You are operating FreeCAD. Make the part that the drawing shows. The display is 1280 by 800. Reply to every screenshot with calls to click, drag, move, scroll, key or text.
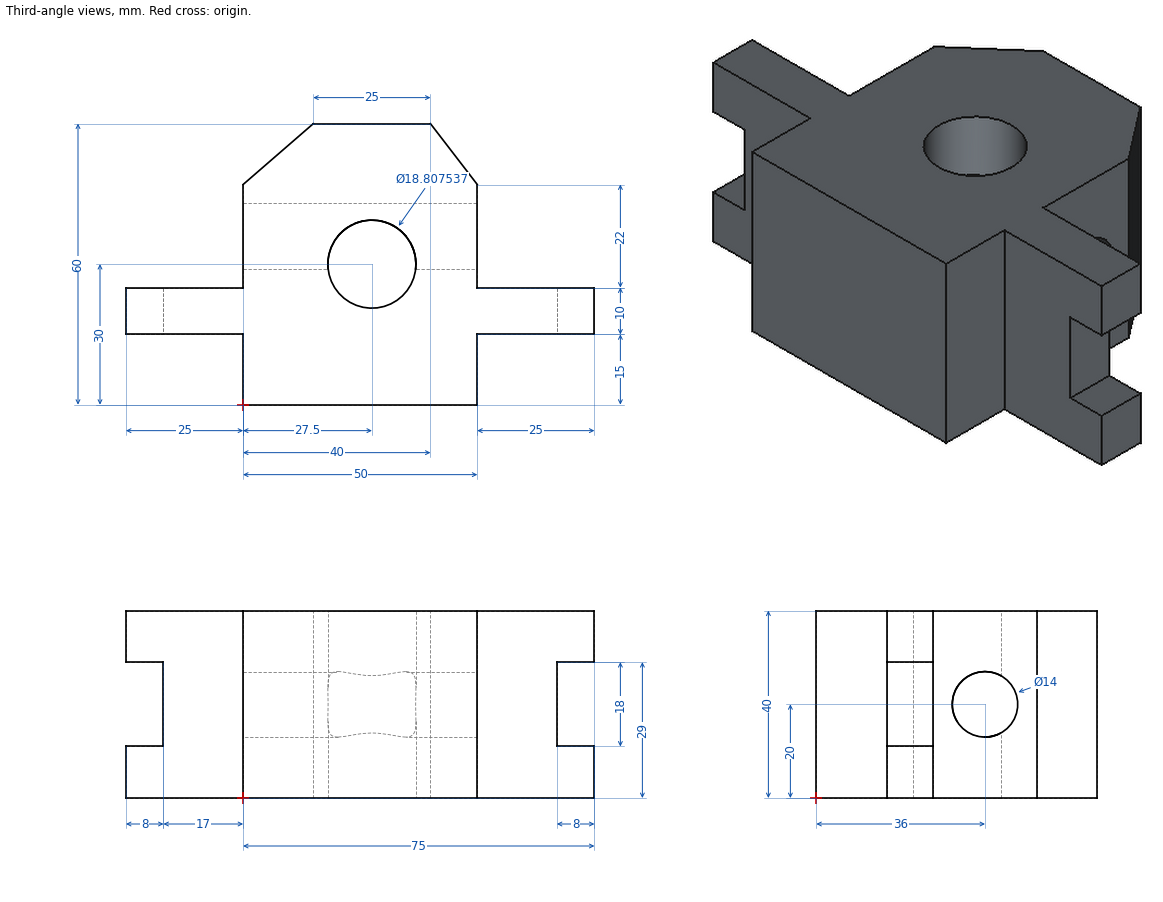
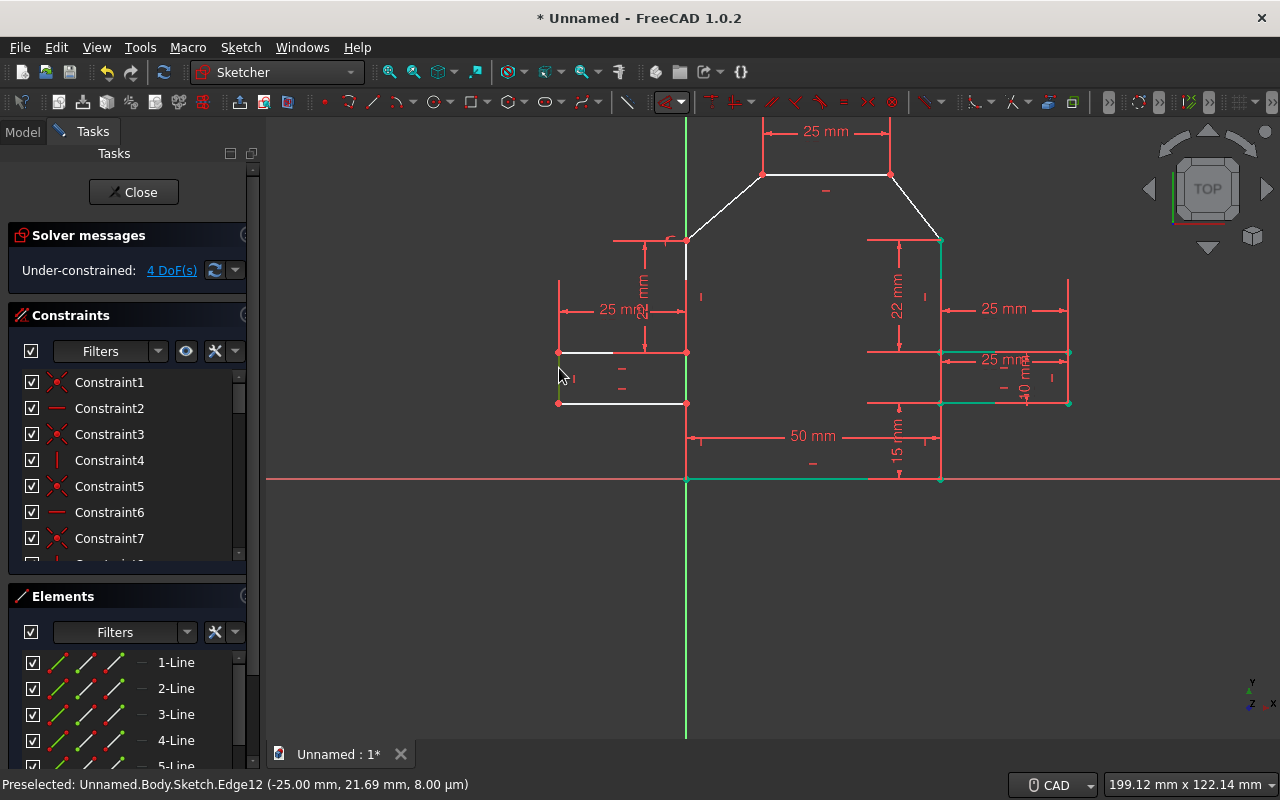
key(i)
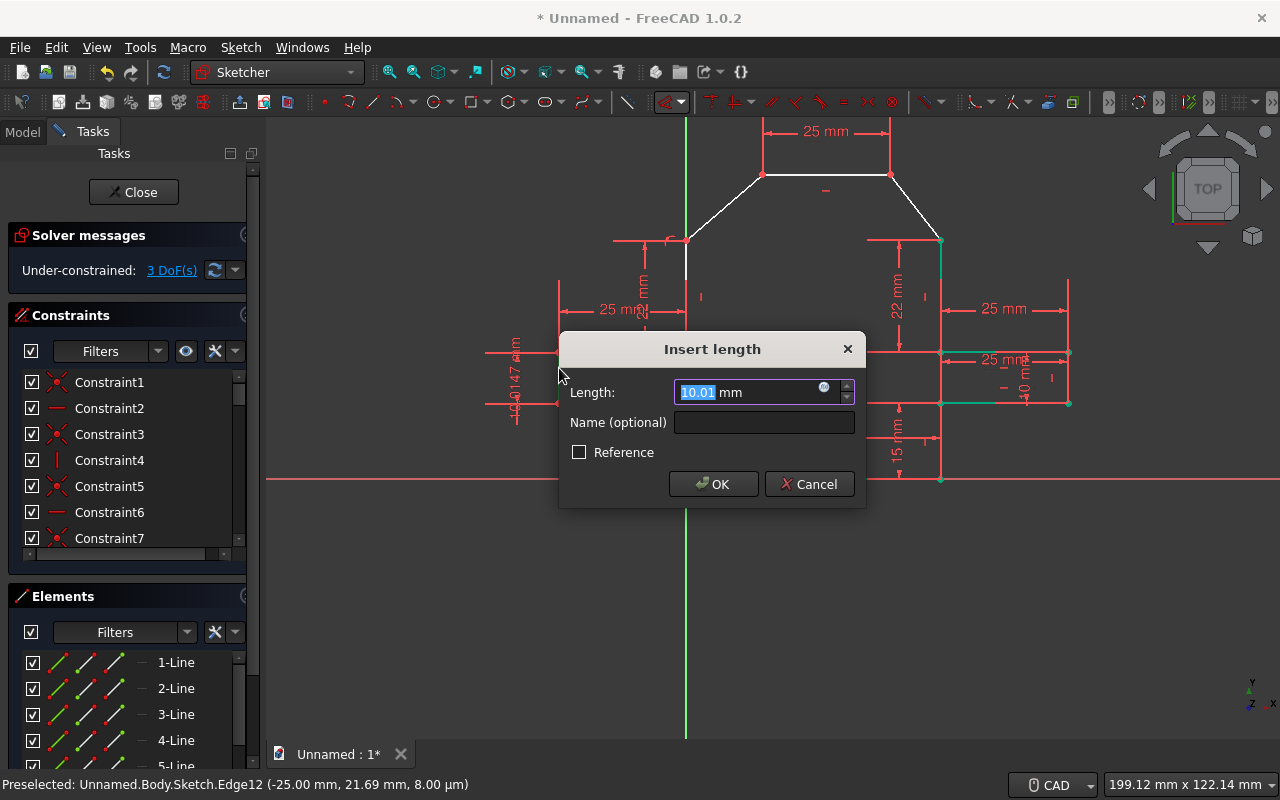
text(10)
key(Return)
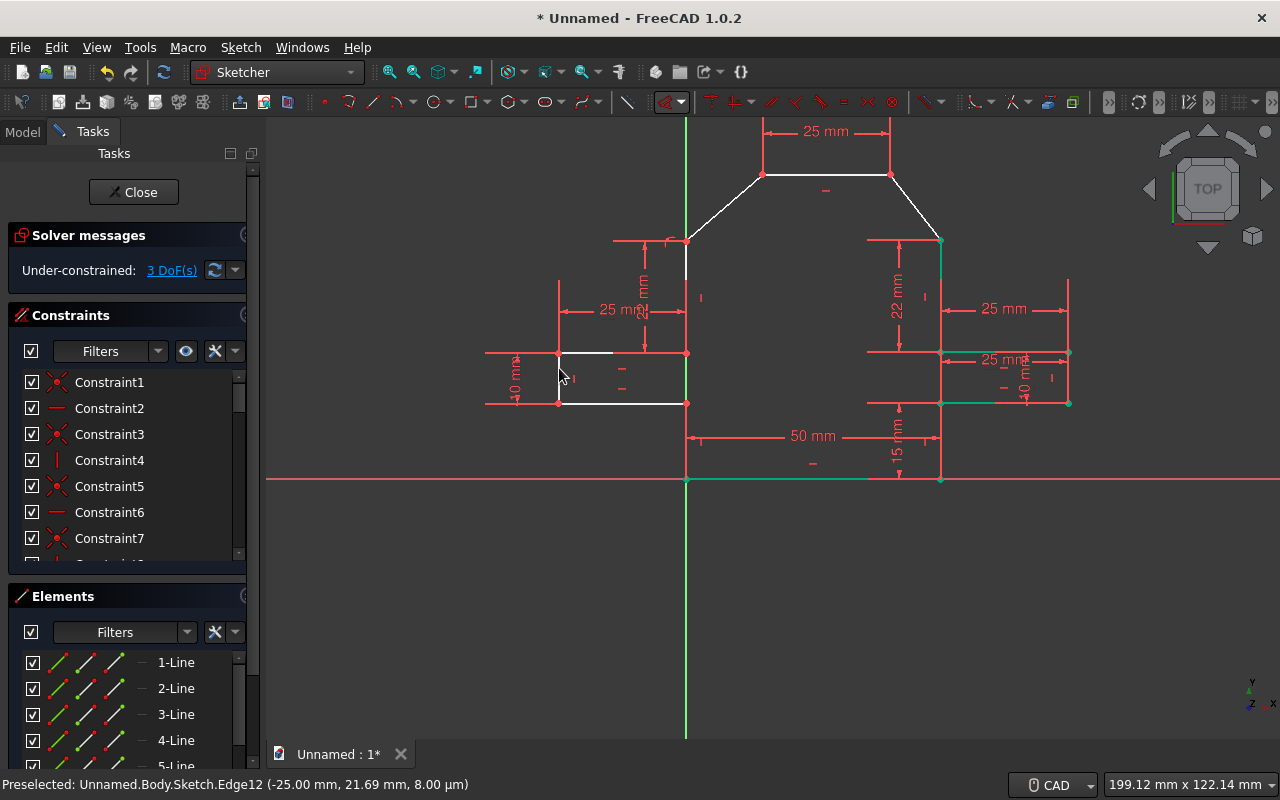
click(686, 427)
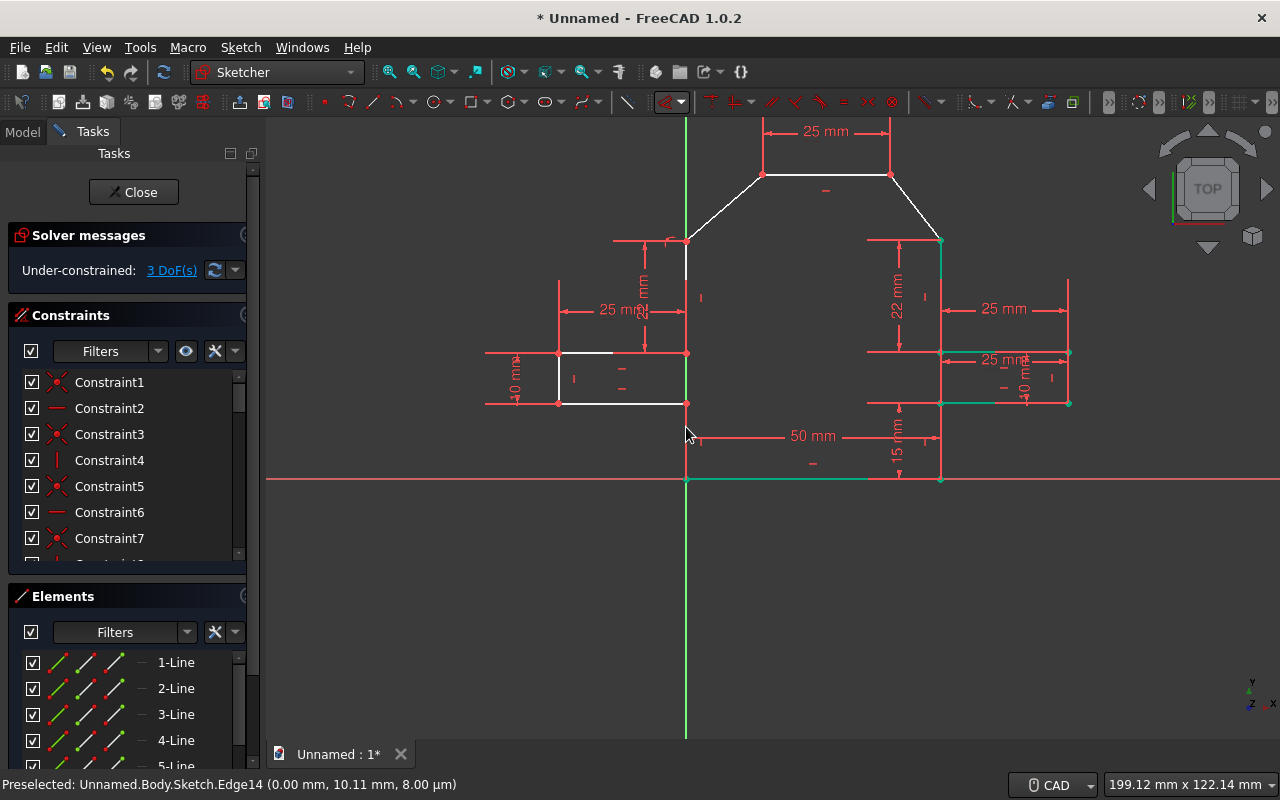
key(i)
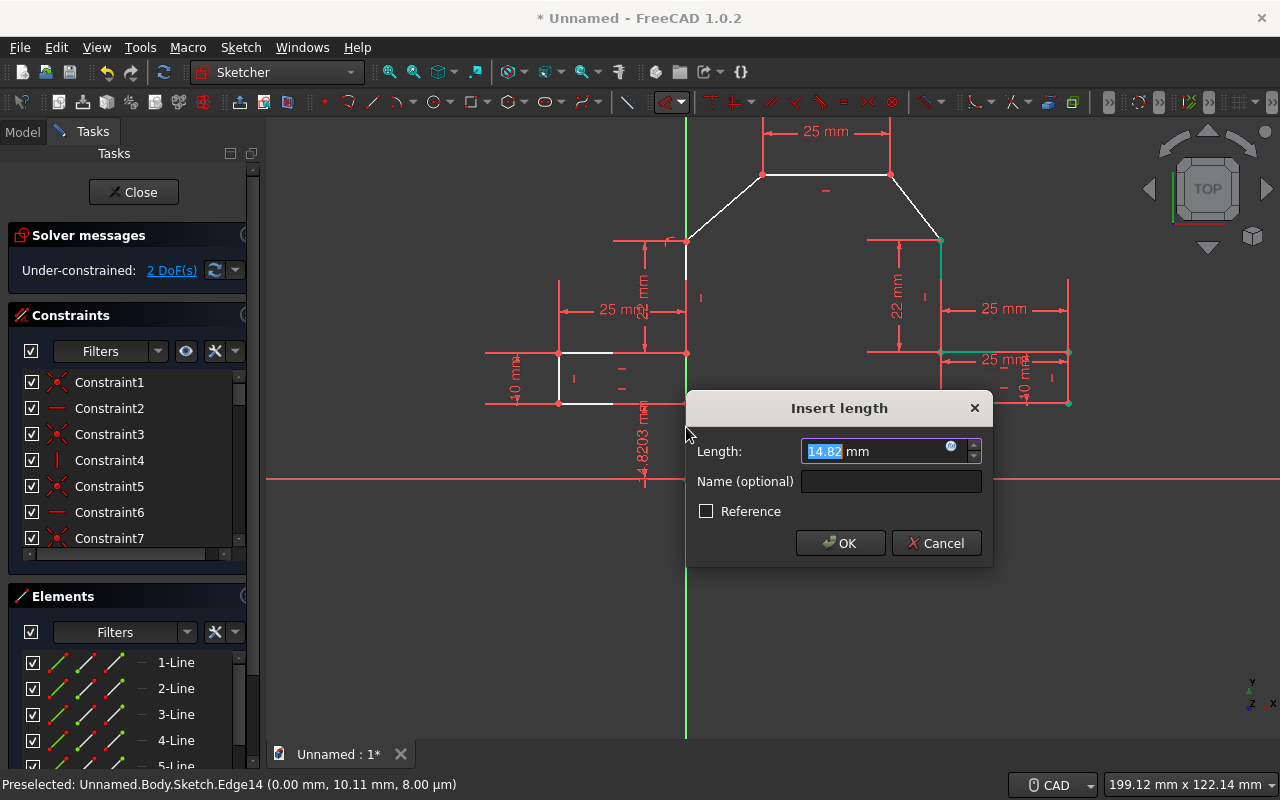
text(15)
key(Return)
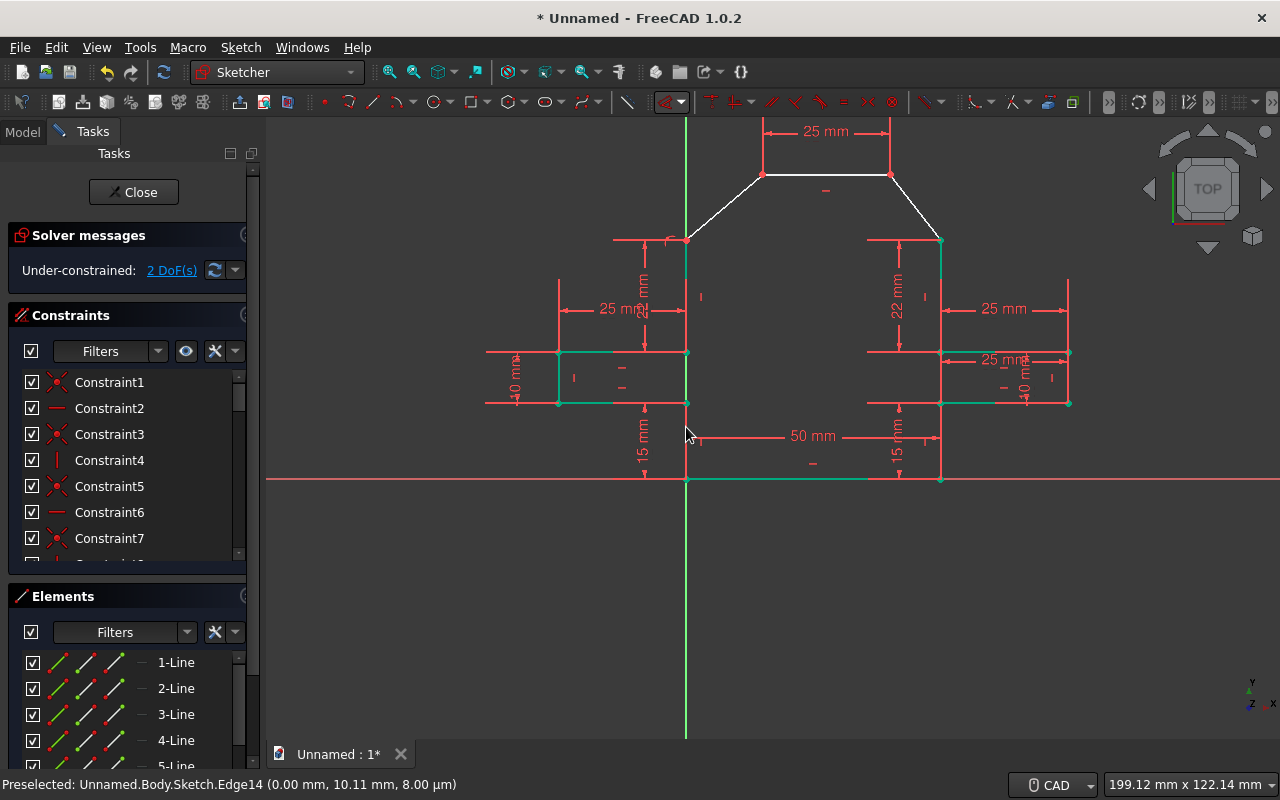
click(890, 175)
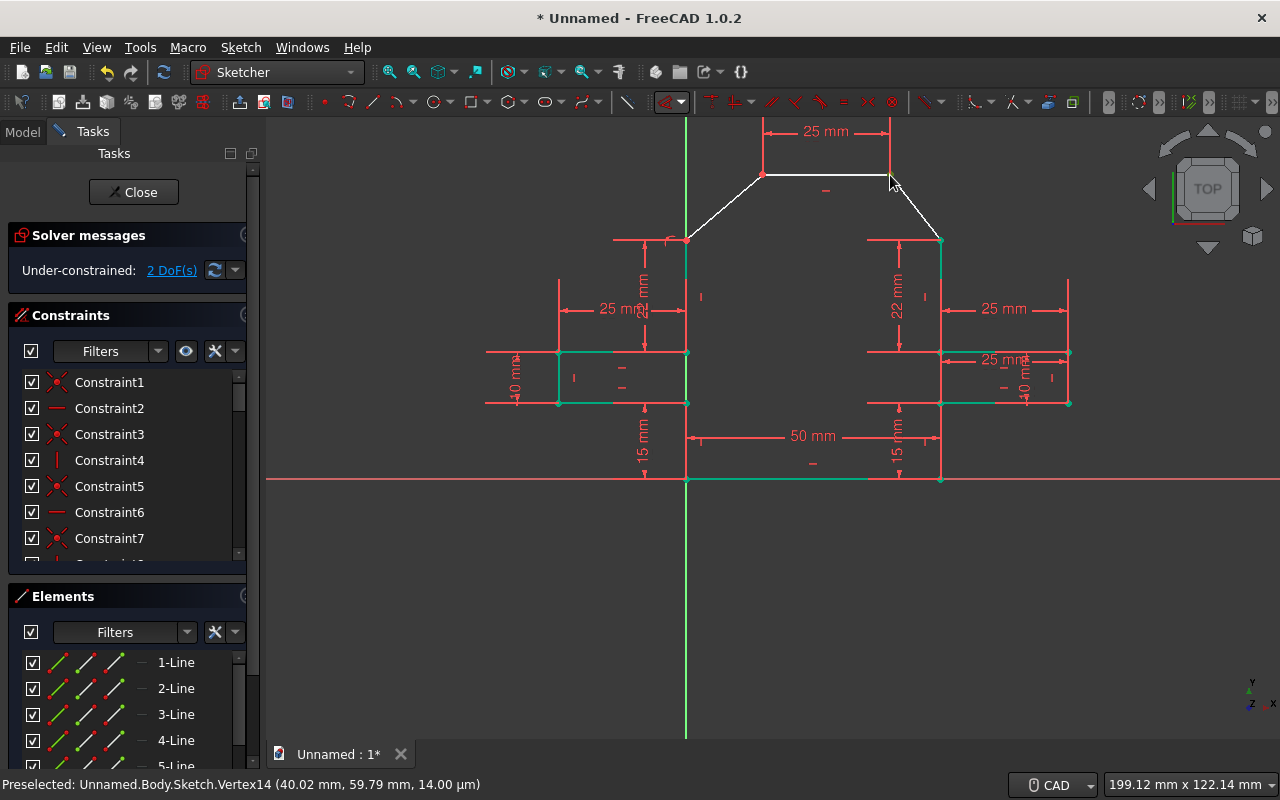
key(l)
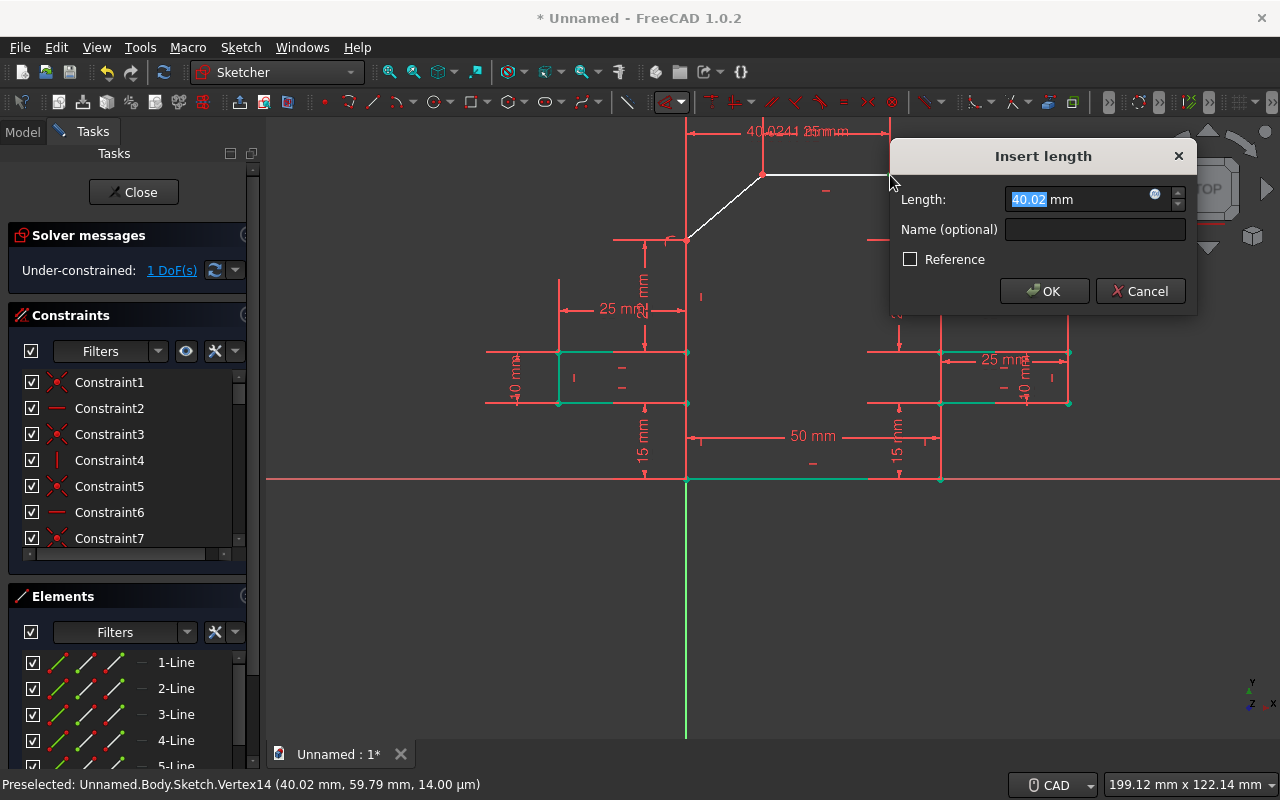
text(40)
key(Return)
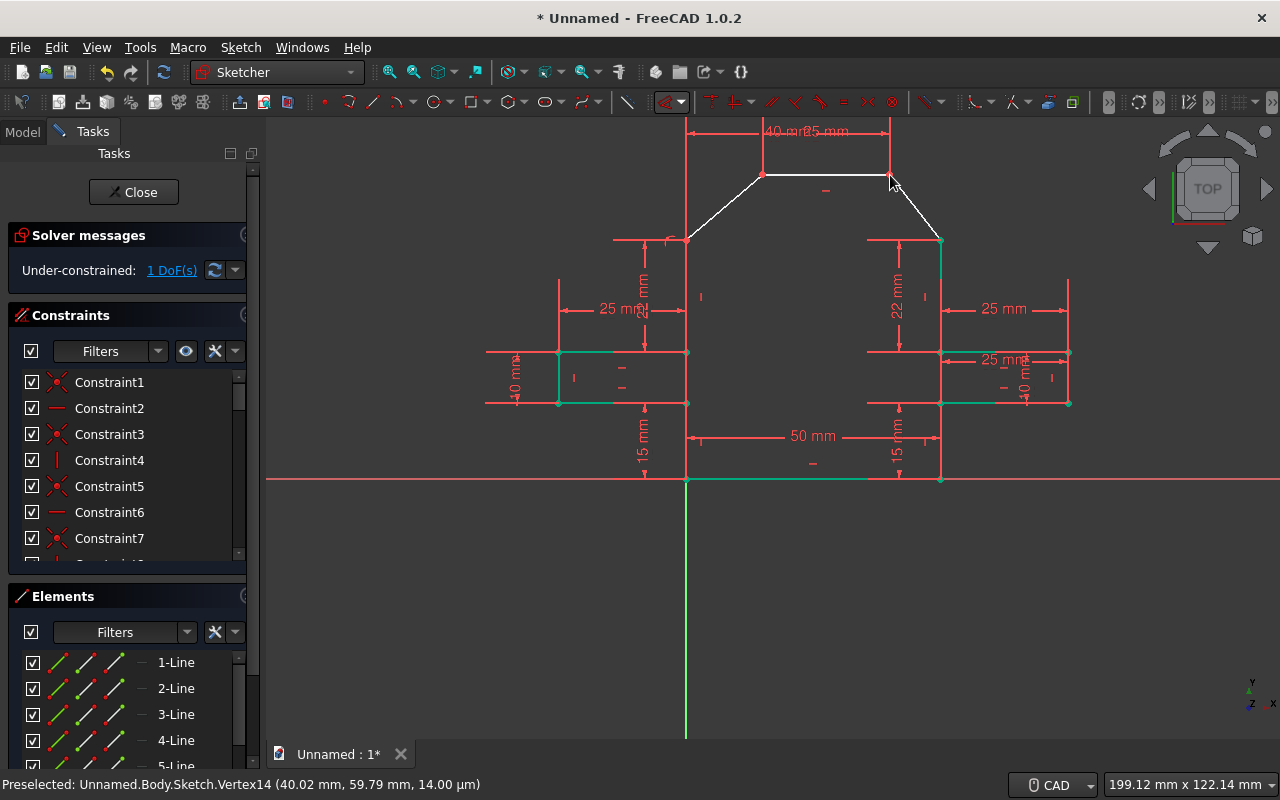
click(890, 175)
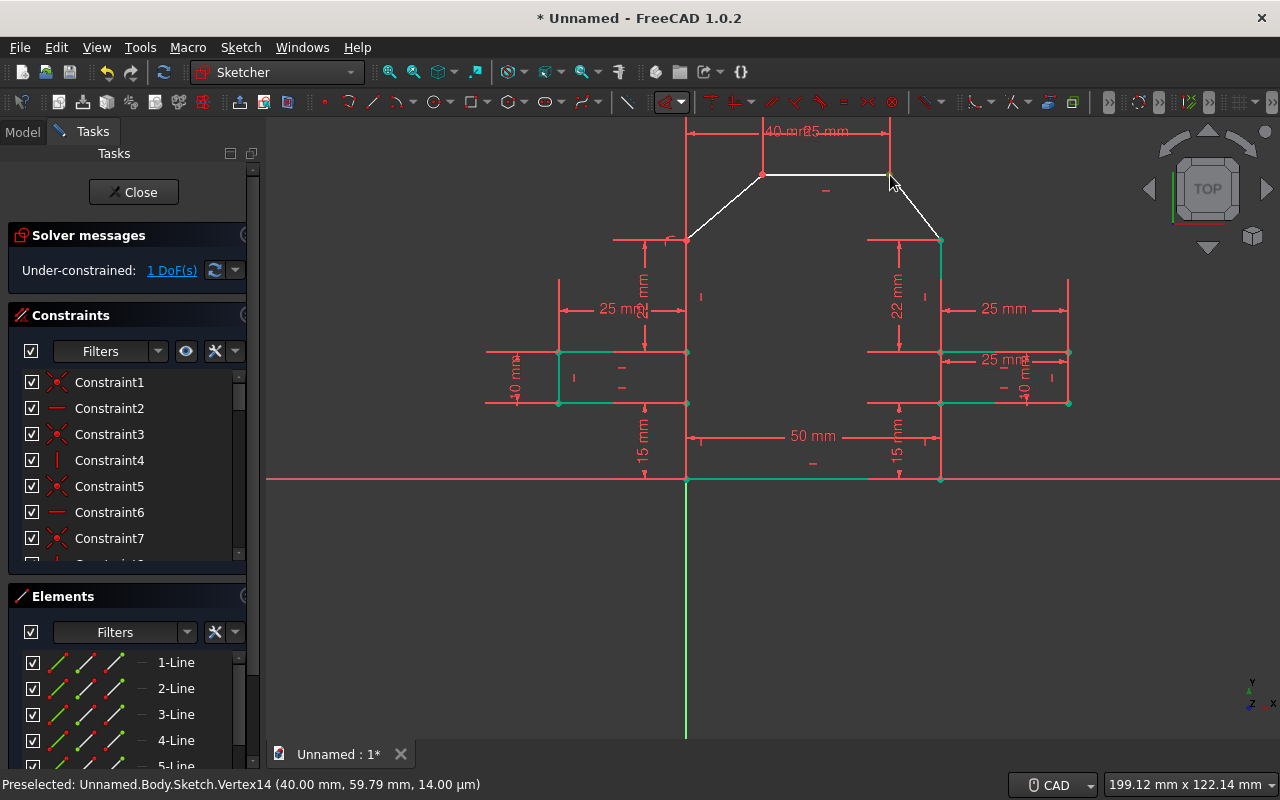
key(i)